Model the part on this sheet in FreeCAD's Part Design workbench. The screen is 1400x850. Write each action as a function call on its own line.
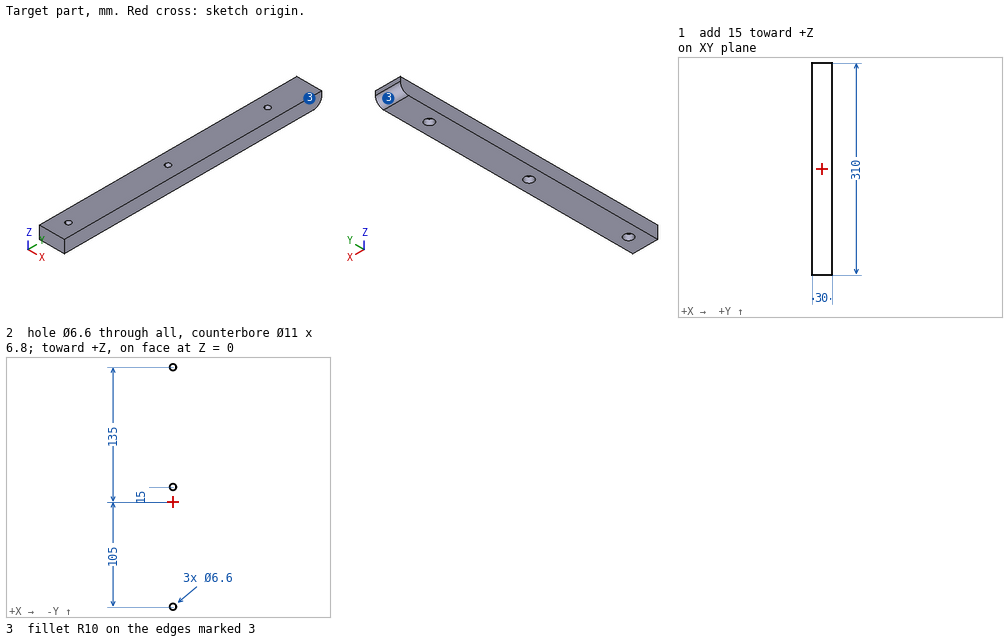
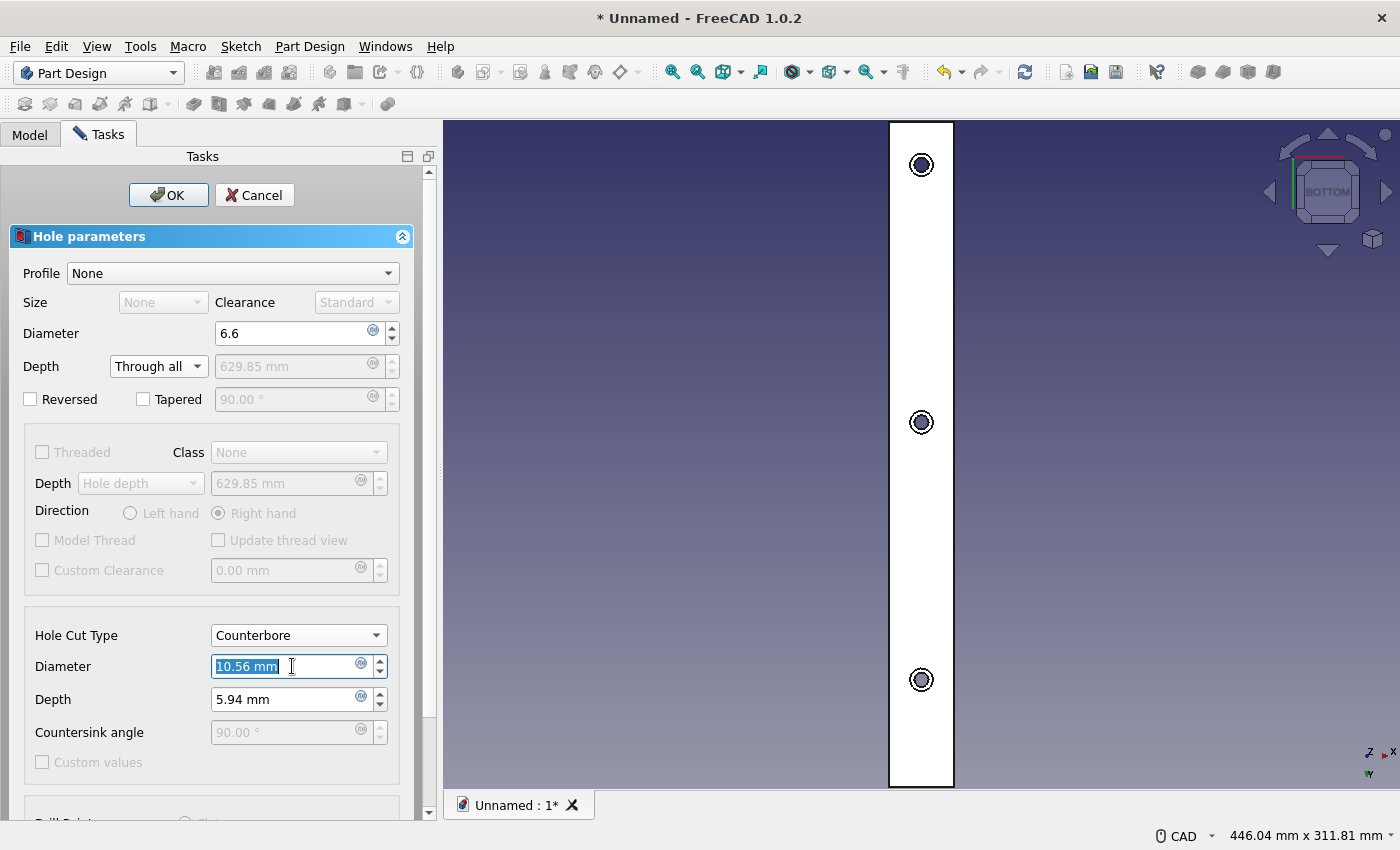
text(11)
key(Tab)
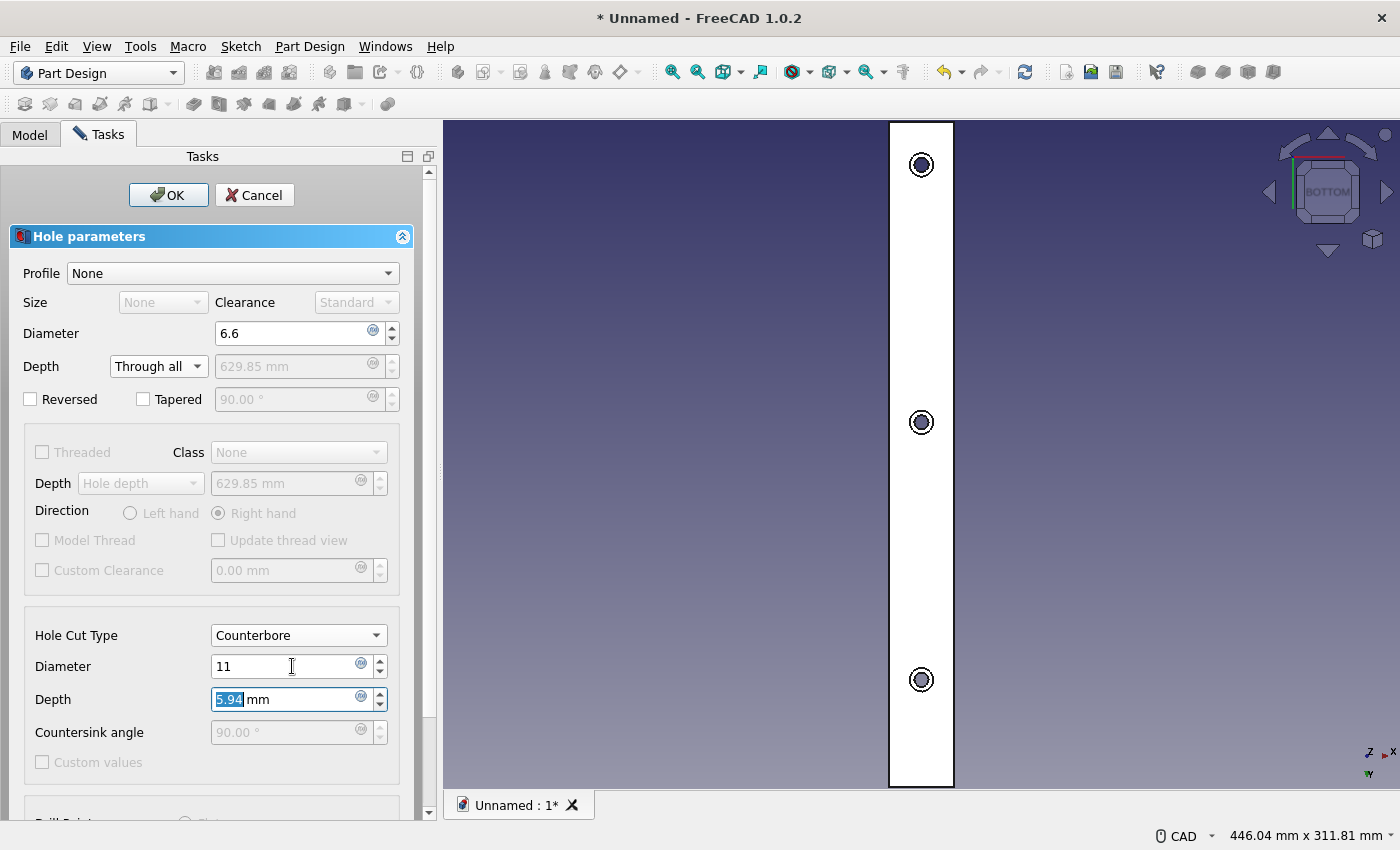
text(6.8)
key(Tab)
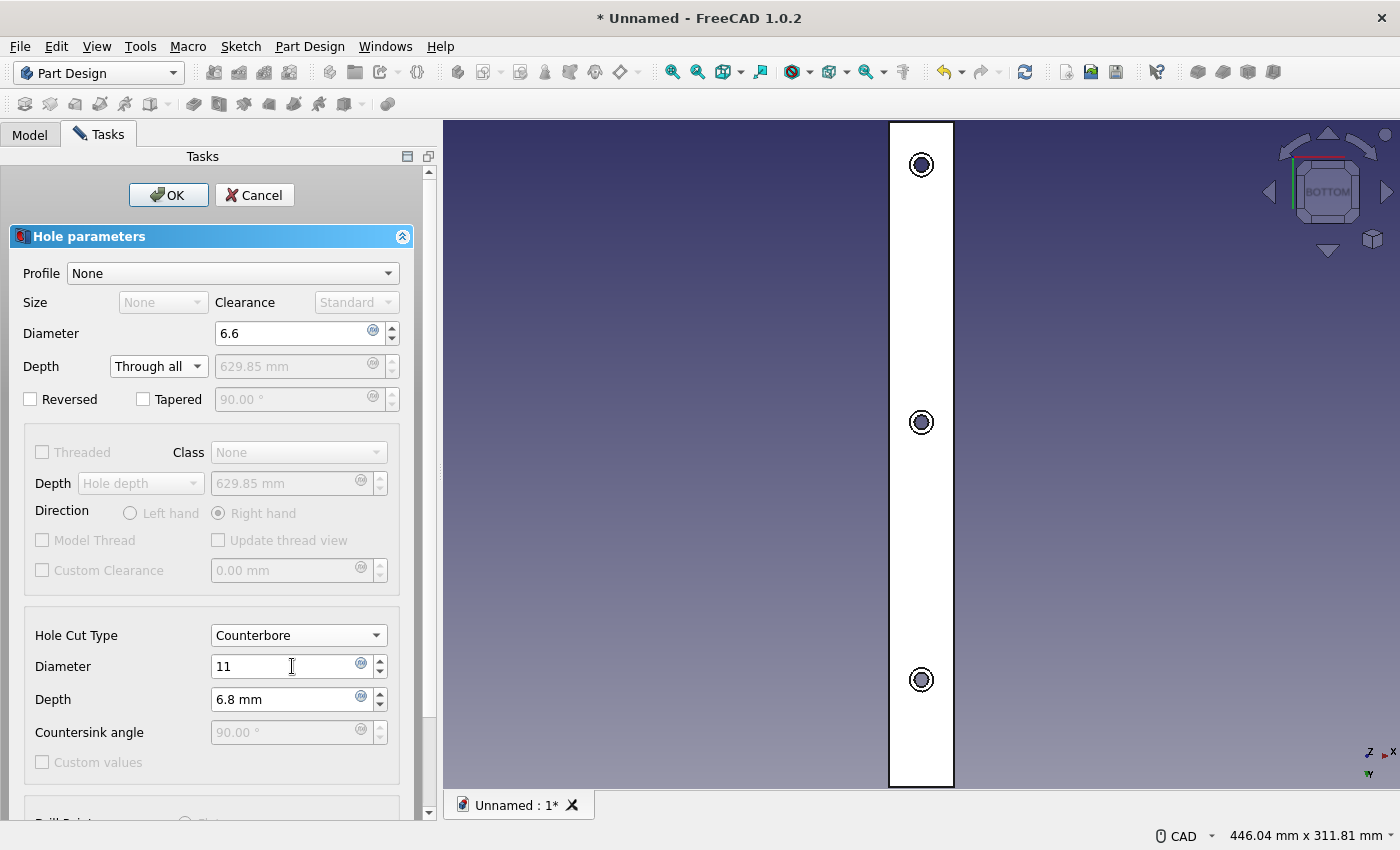
click(169, 195)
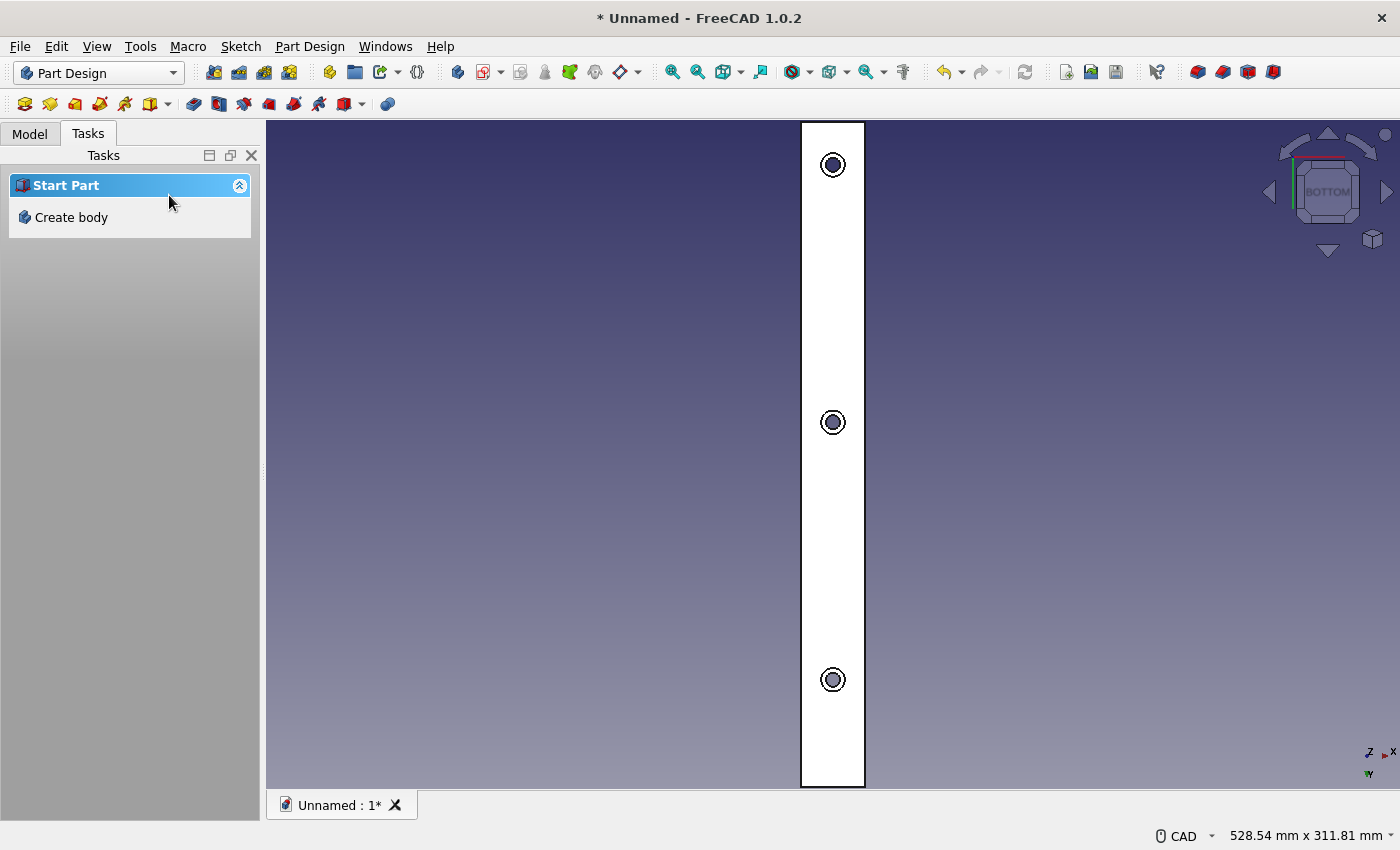
key(0)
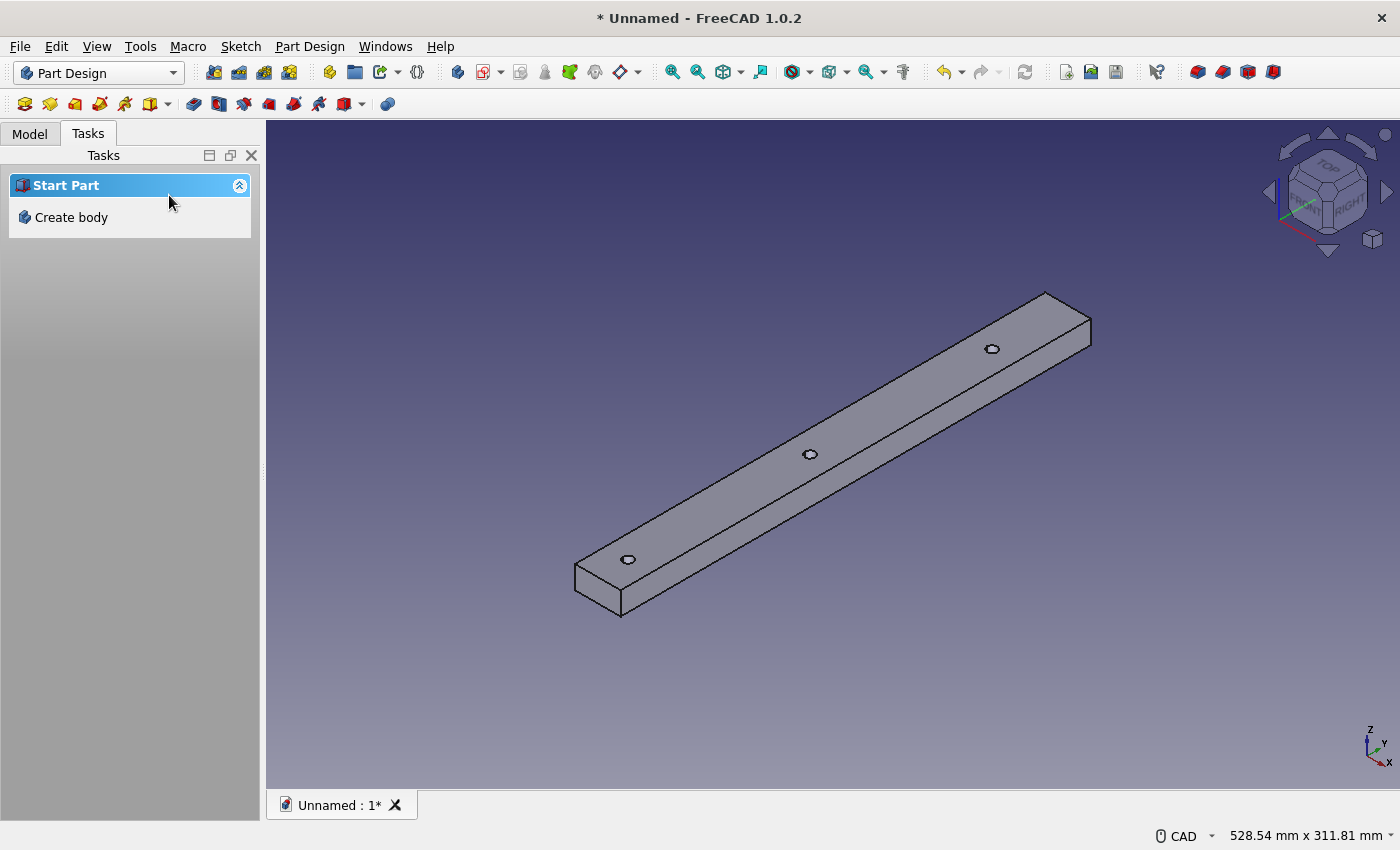
key(2)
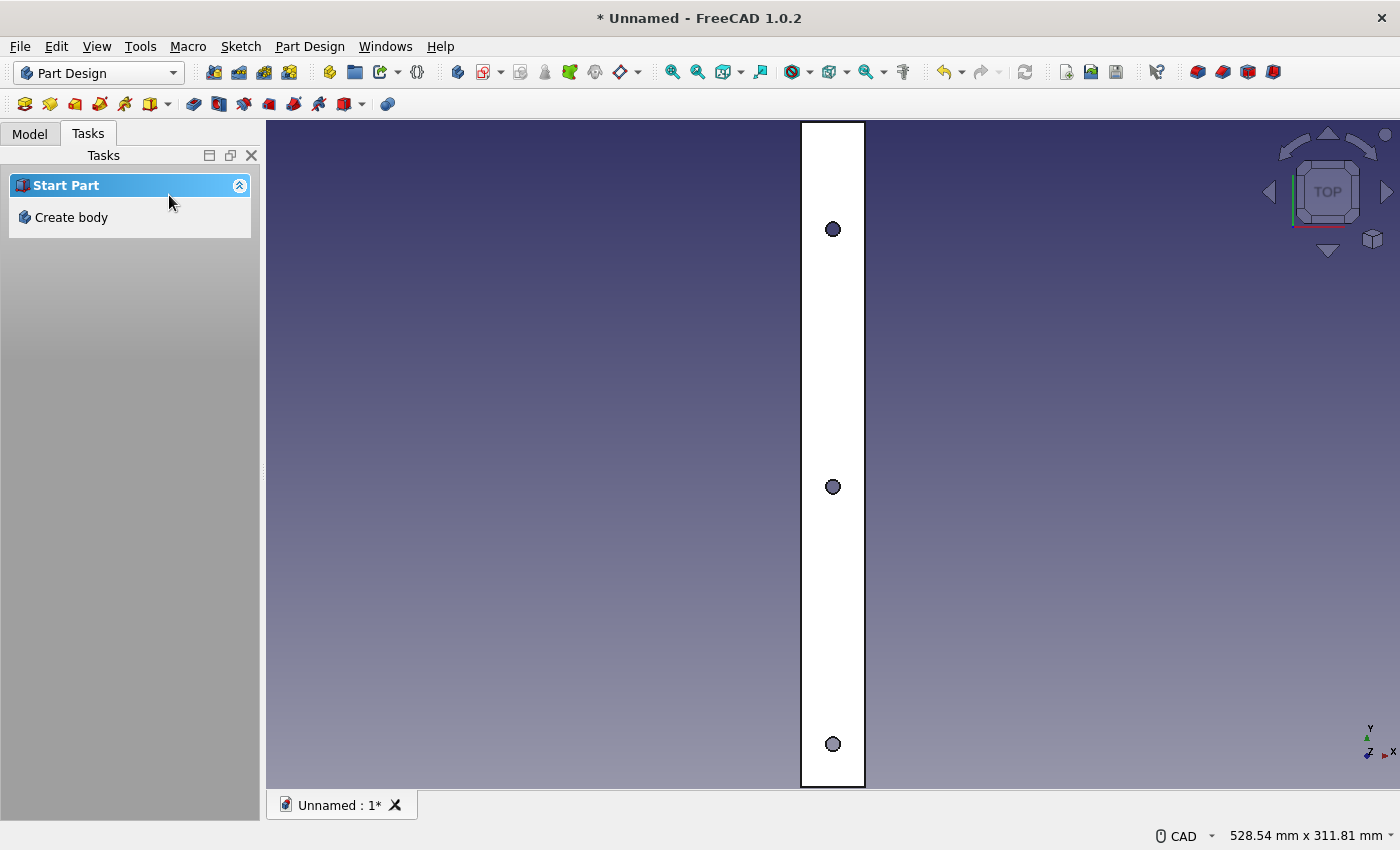
key(1)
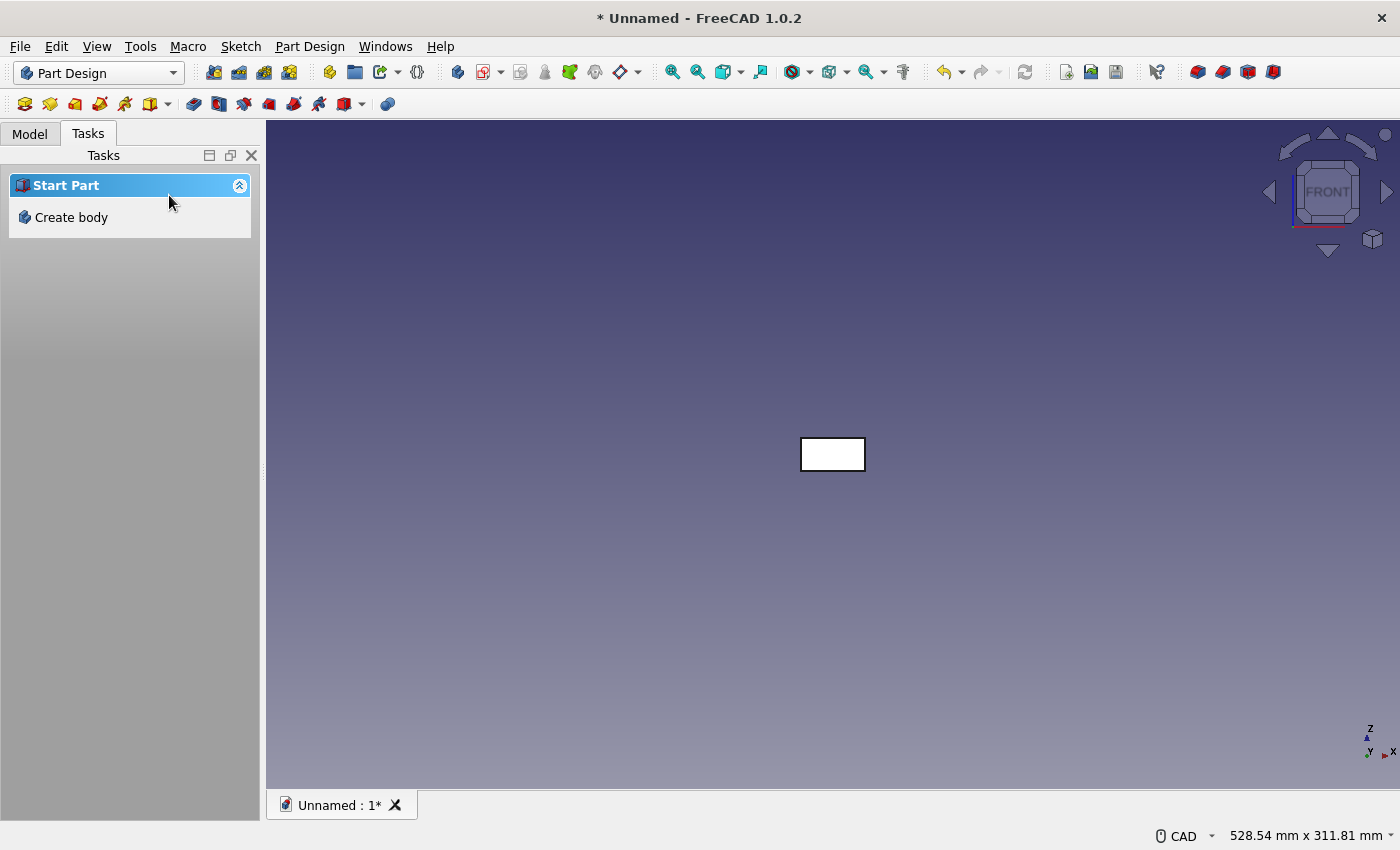
click(673, 72)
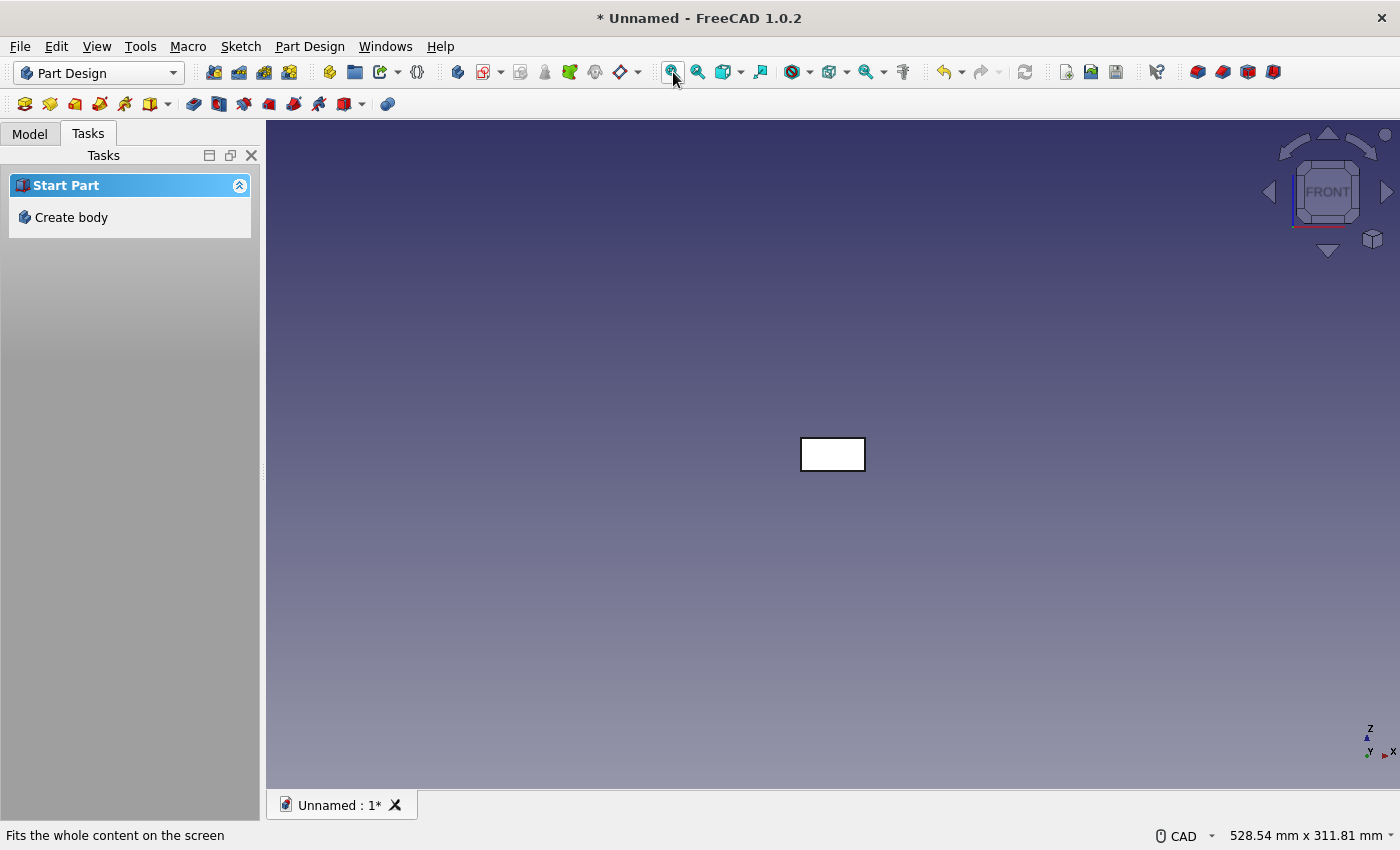
key(3)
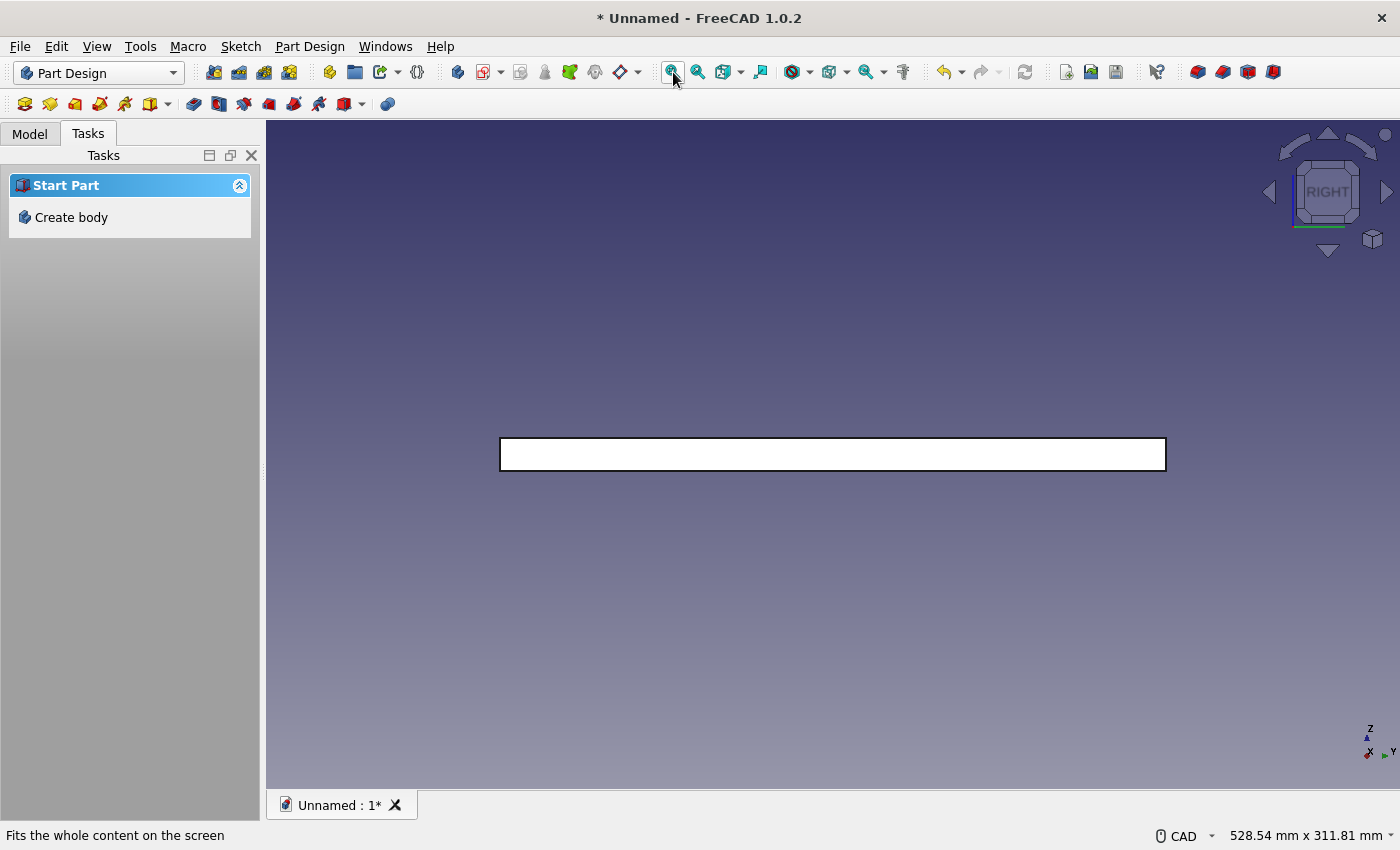
key(5)